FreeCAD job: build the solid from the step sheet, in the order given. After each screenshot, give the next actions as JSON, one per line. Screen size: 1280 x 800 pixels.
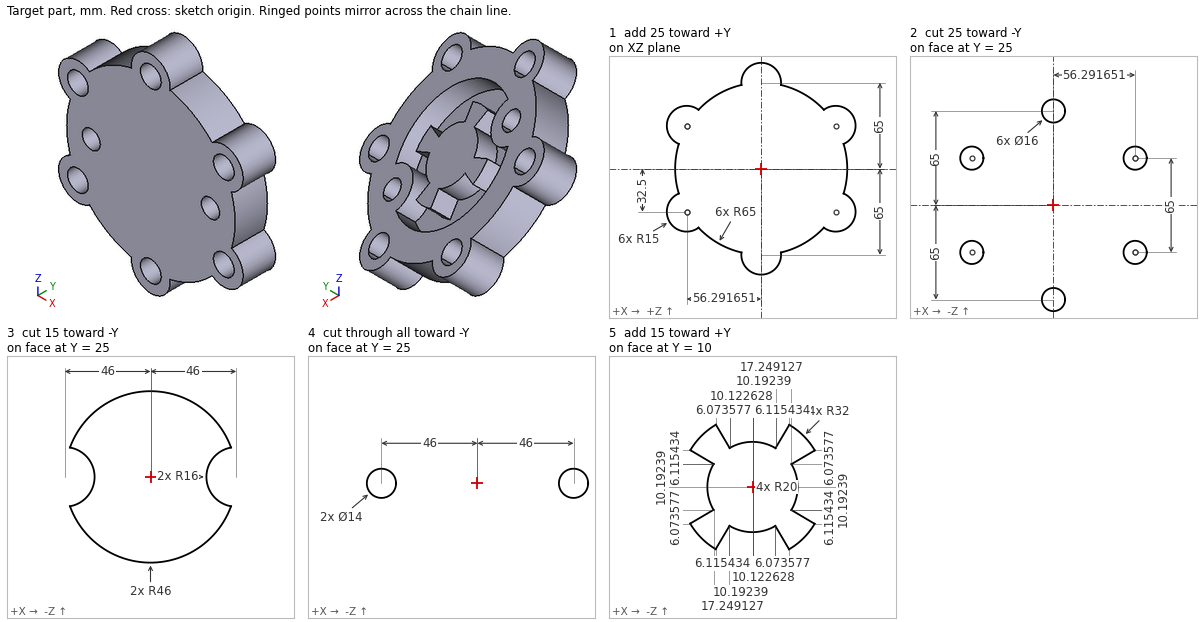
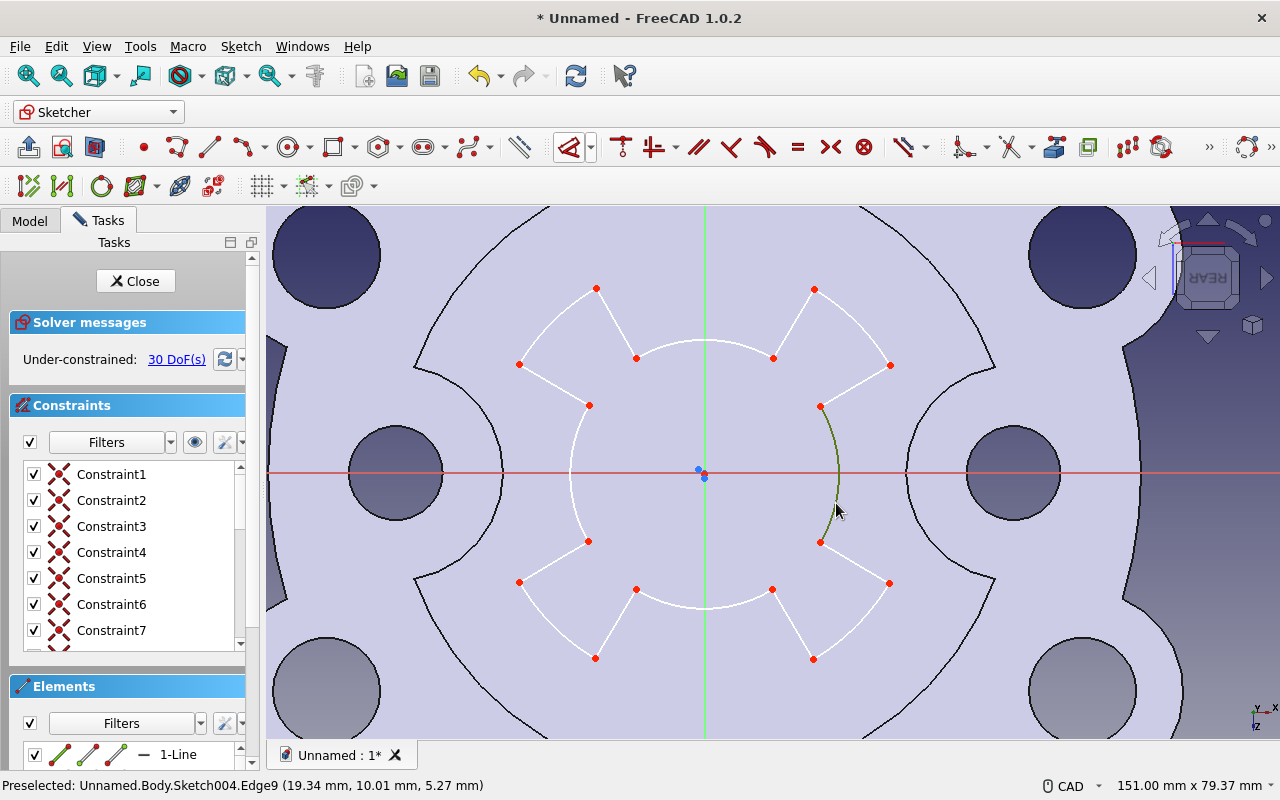
{"action": "left_click", "coordinate": [676, 606]}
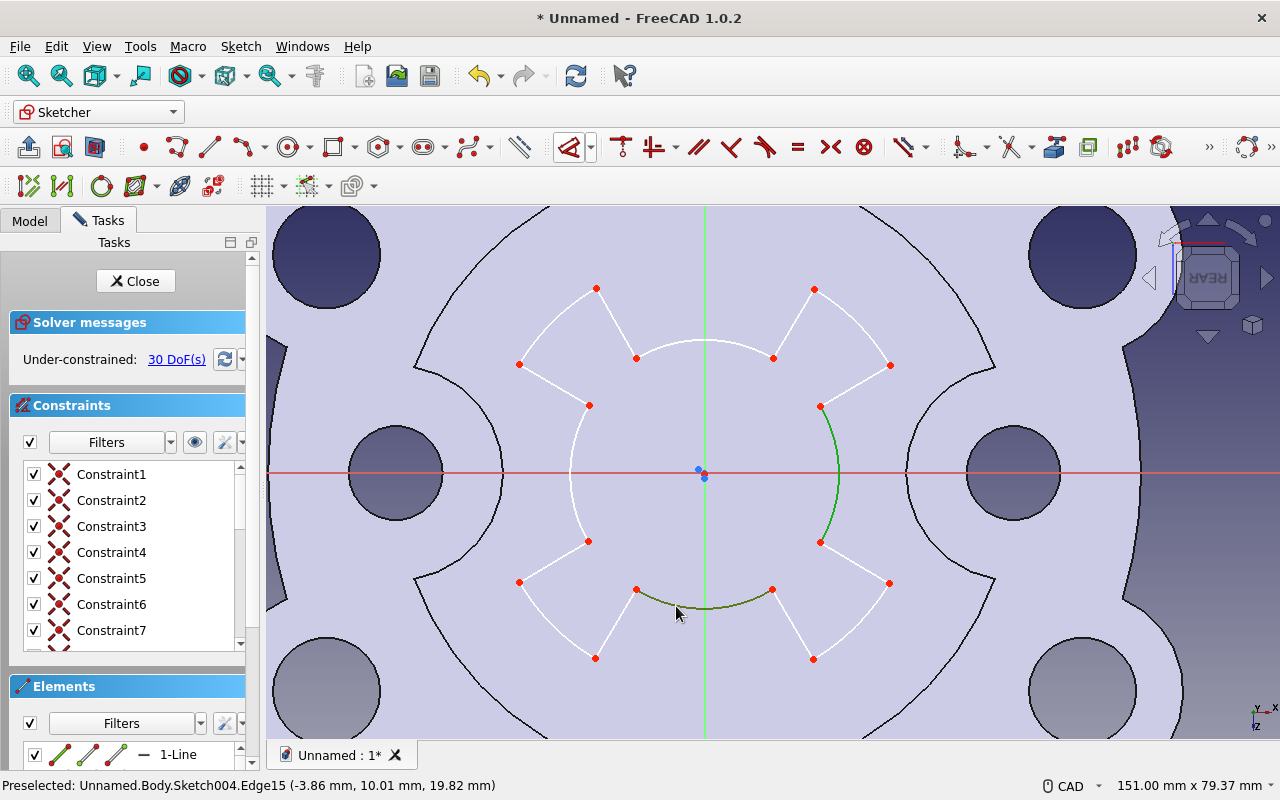
{"action": "left_click", "coordinate": [621, 148]}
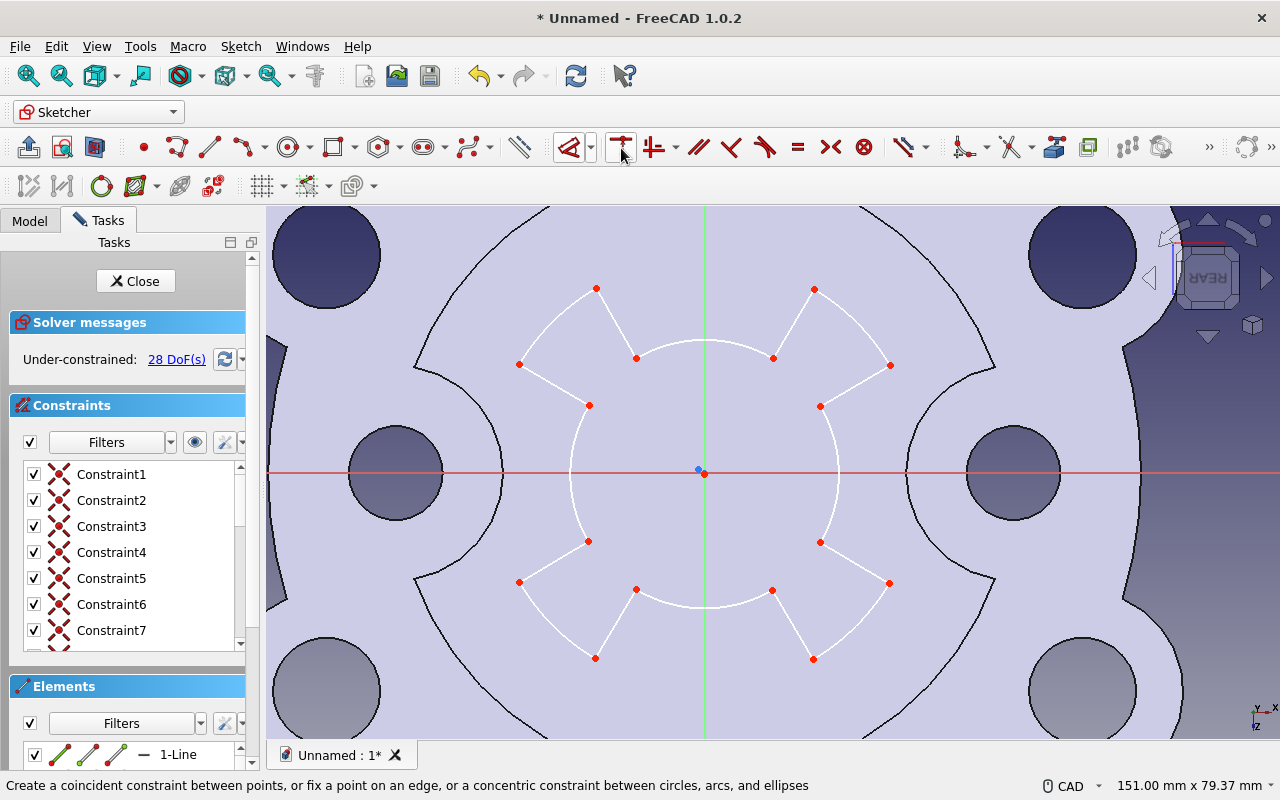
{"action": "left_click", "coordinate": [836, 503]}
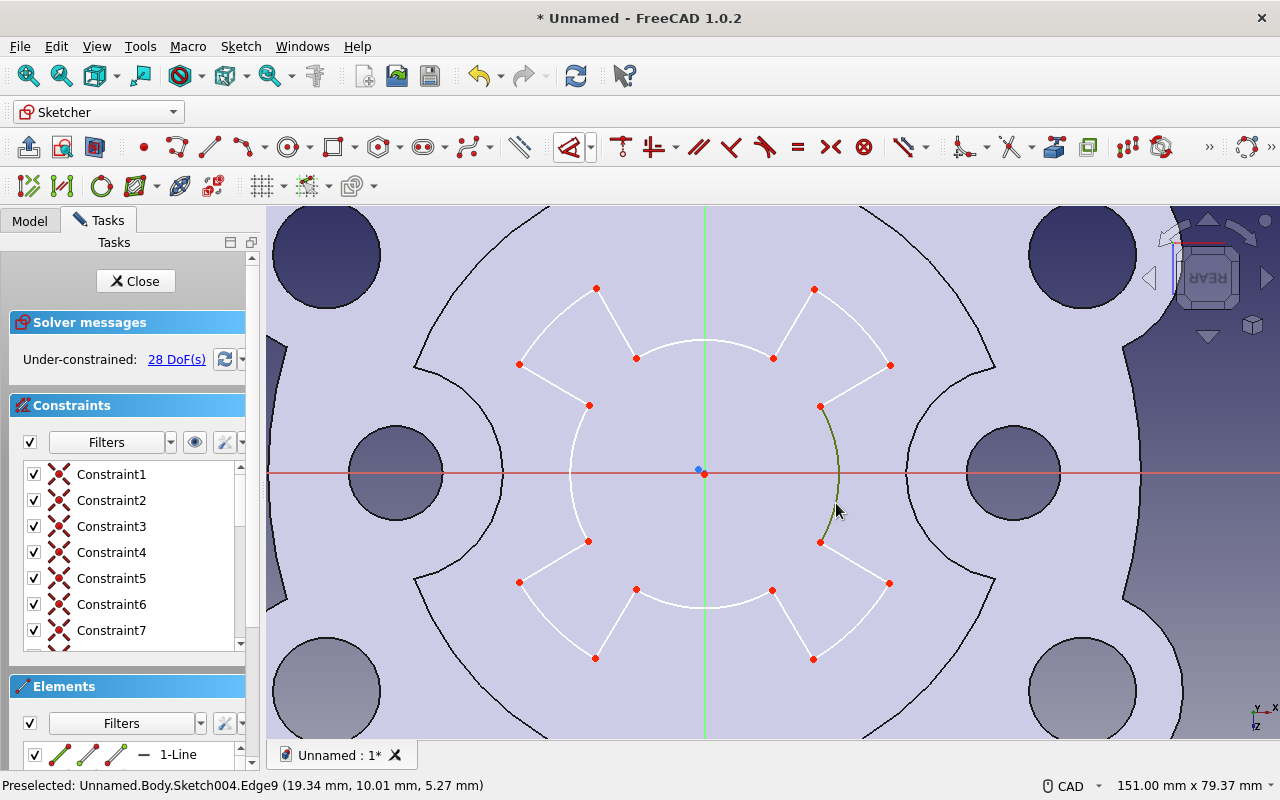
{"action": "left_click", "coordinate": [840, 641]}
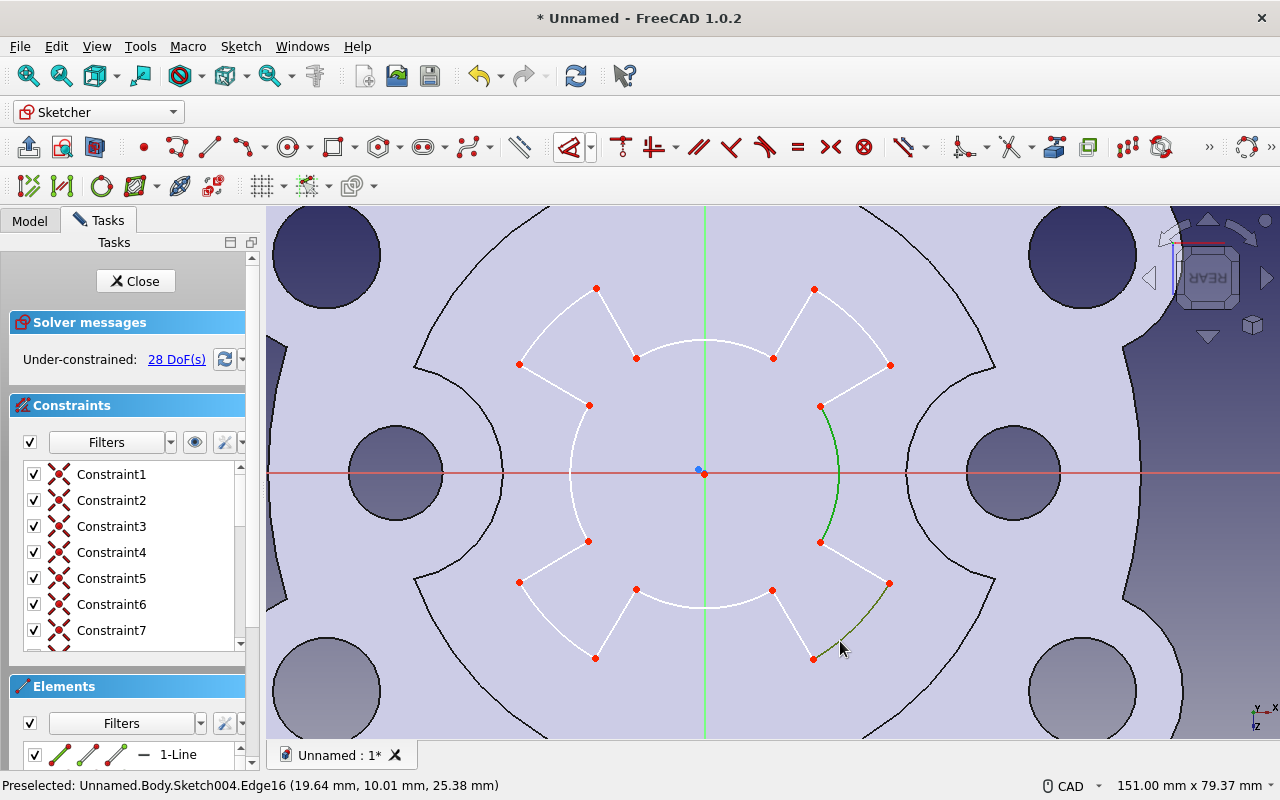
{"action": "left_click", "coordinate": [621, 148]}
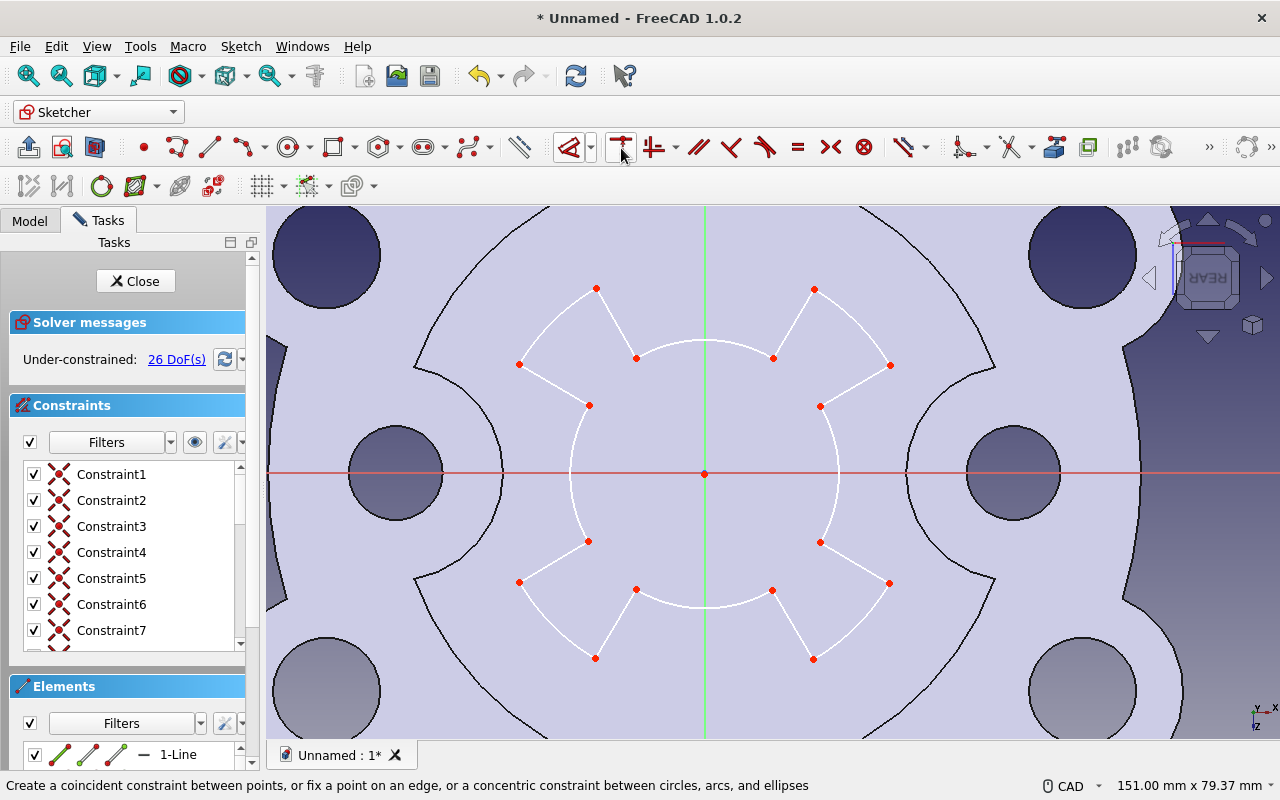
{"action": "left_click_drag", "start_coordinate": [695, 463], "coordinate": [715, 484]}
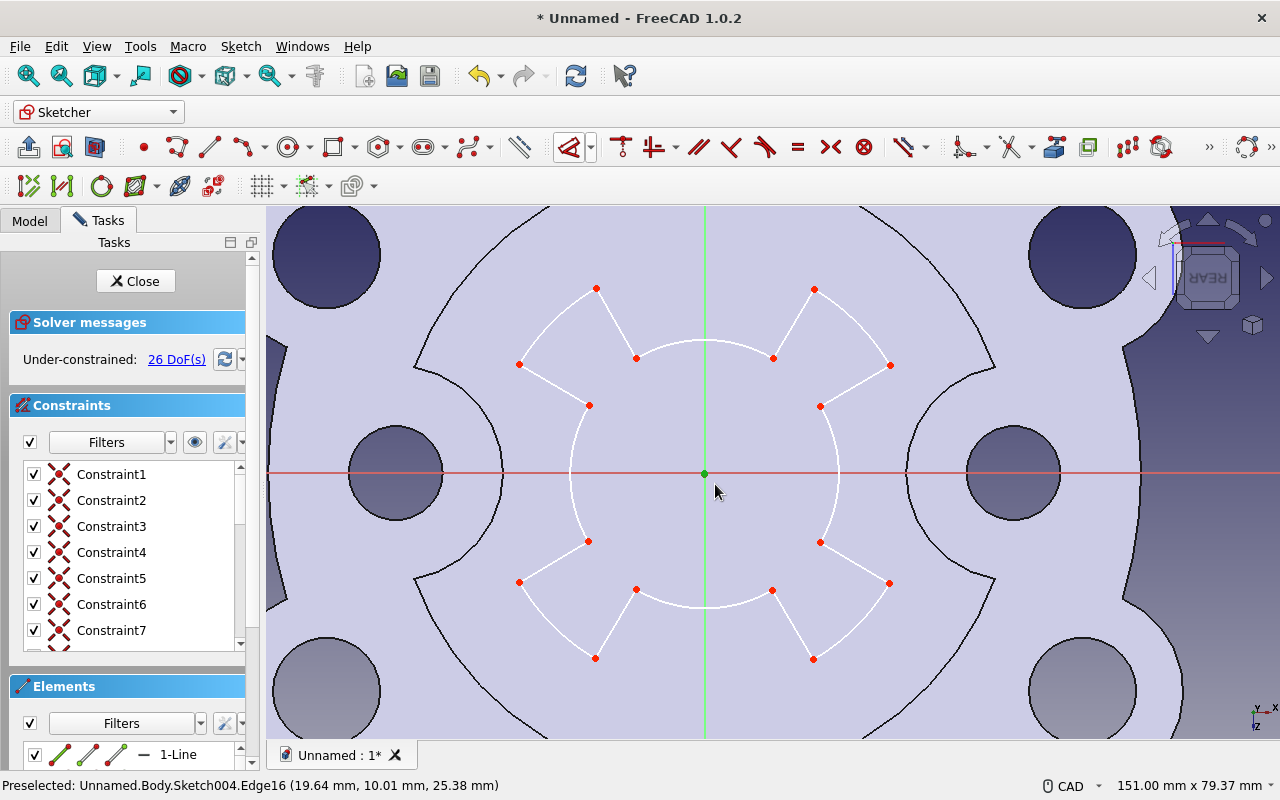
{"action": "key", "text": "c"}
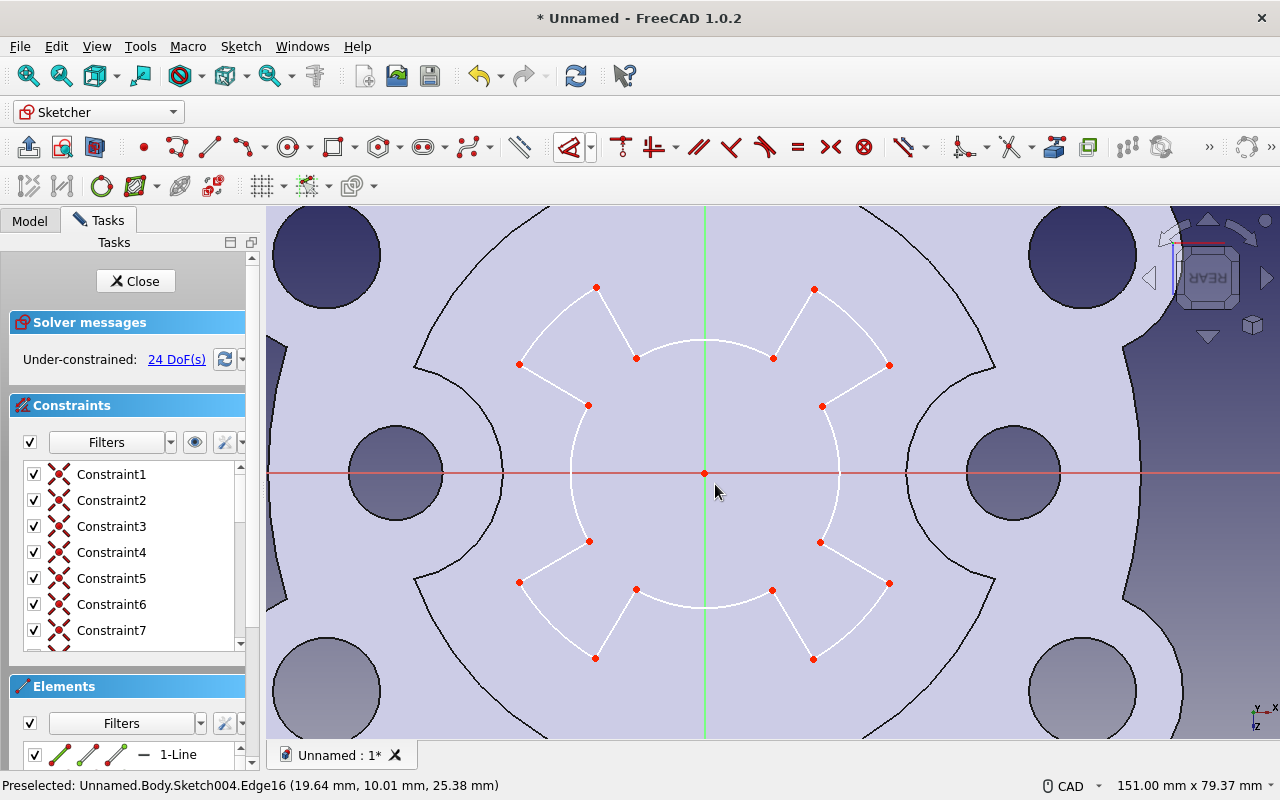
{"action": "left_click", "coordinate": [836, 503]}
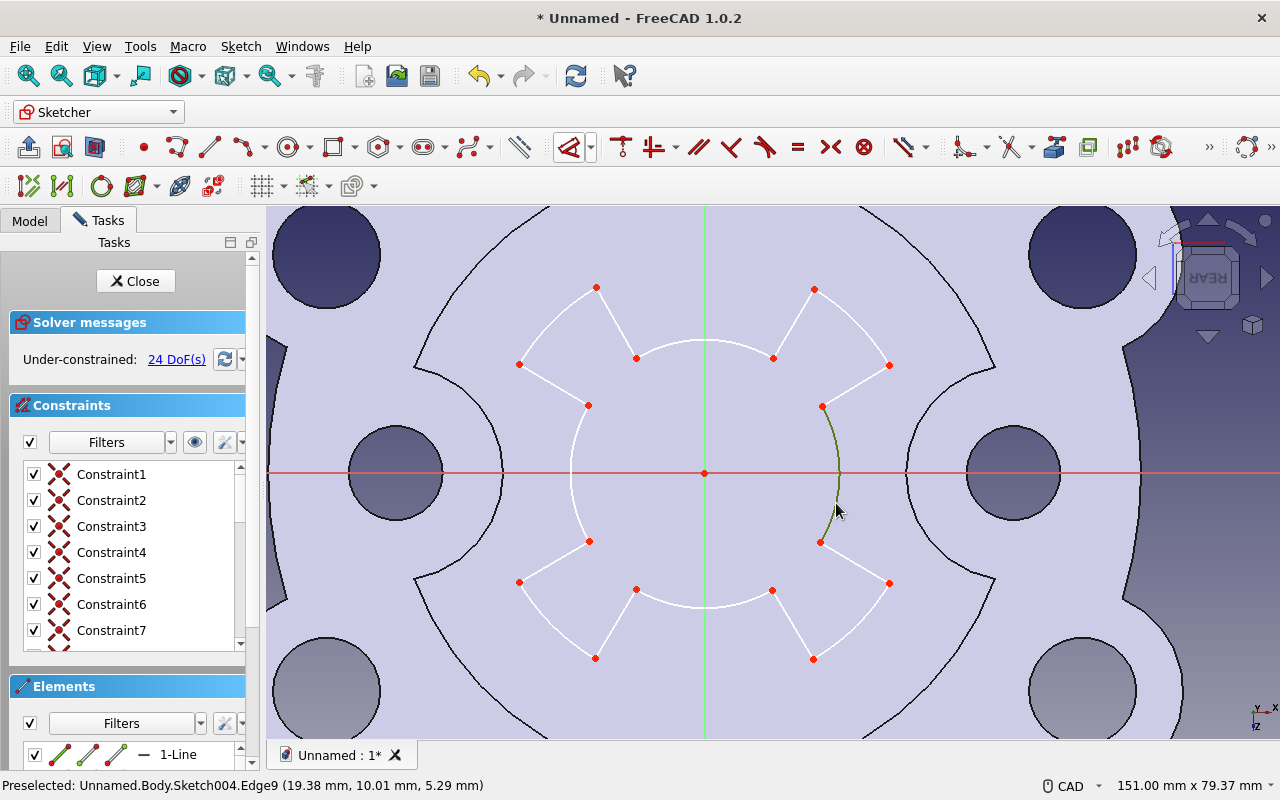
{"action": "left_click", "coordinate": [733, 343]}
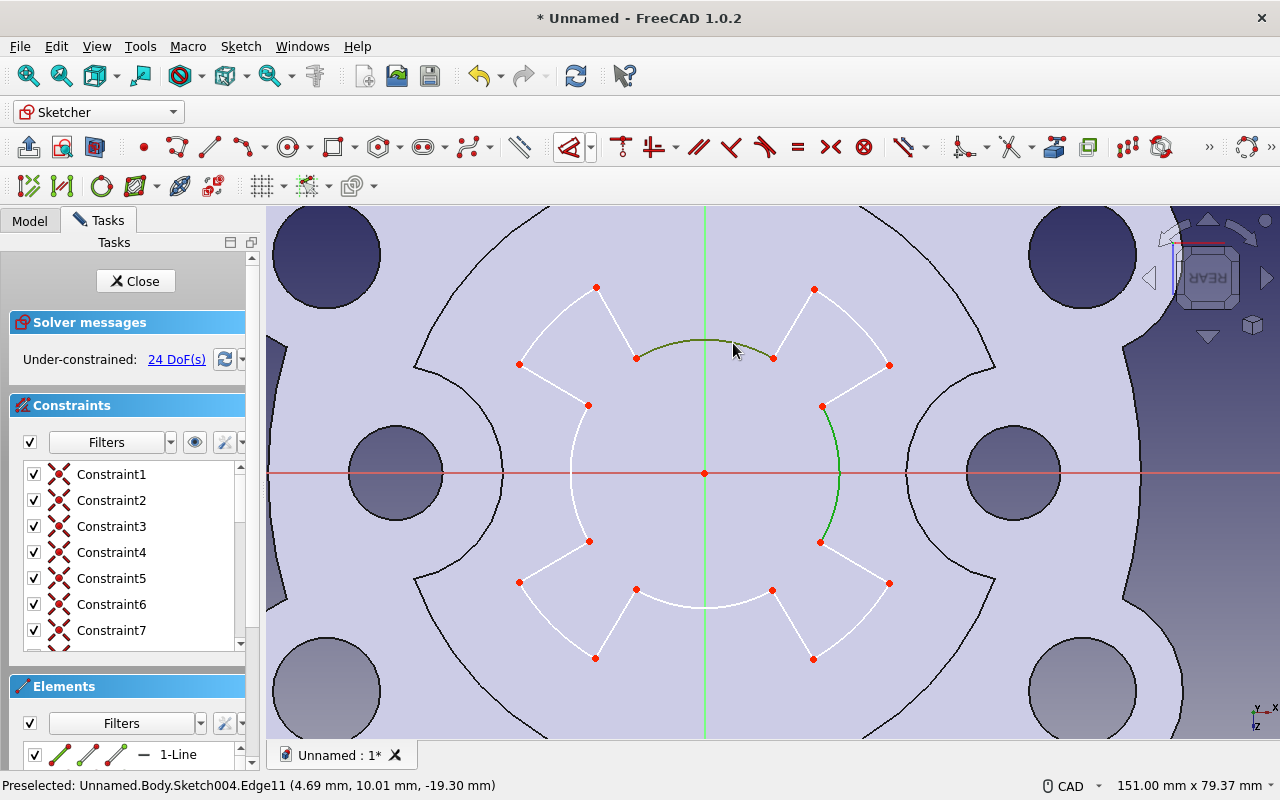
{"action": "left_click", "coordinate": [573, 445]}